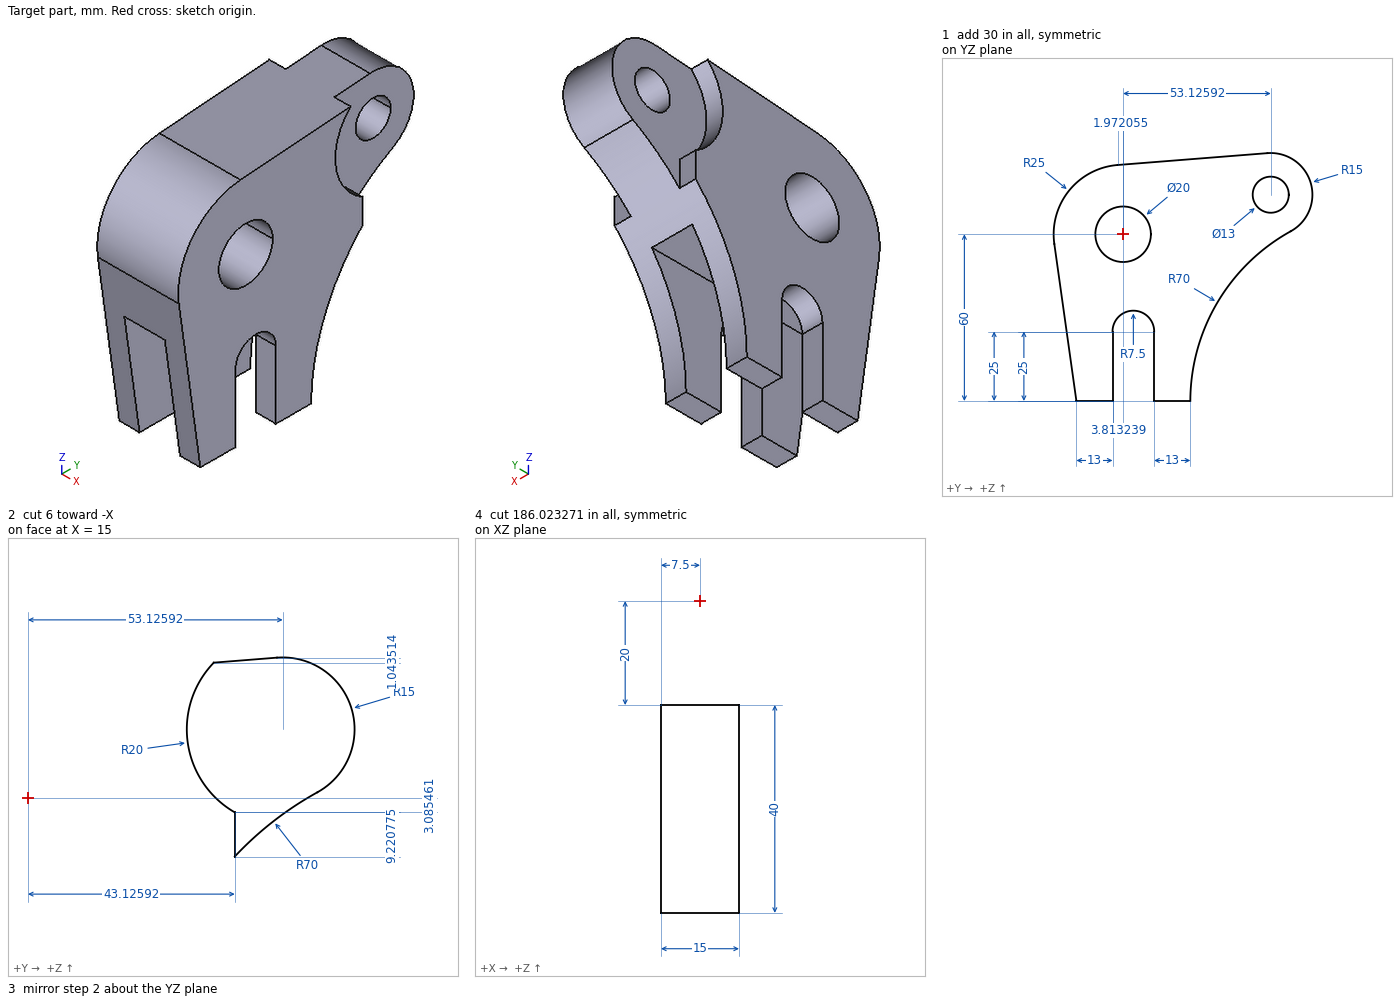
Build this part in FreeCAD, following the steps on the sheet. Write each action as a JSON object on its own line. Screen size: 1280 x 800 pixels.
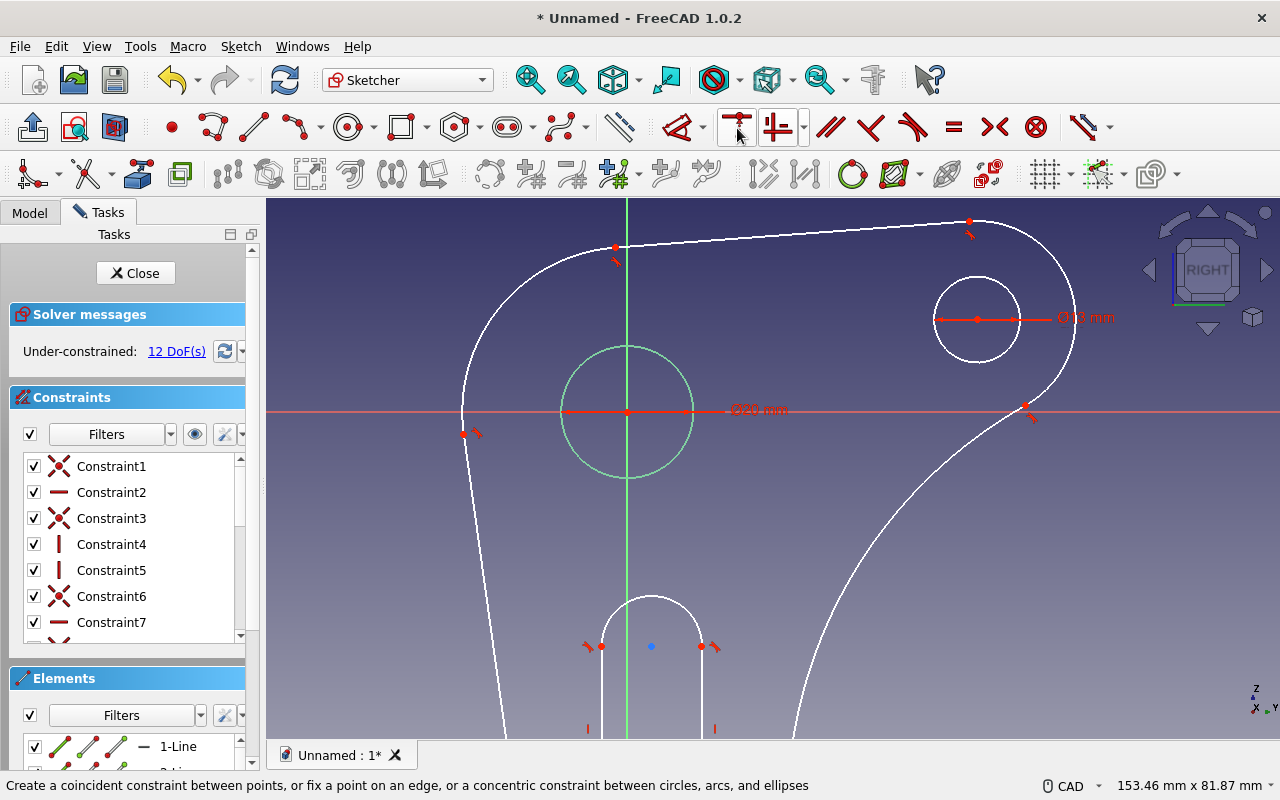
{"action": "left_click", "coordinate": [539, 273]}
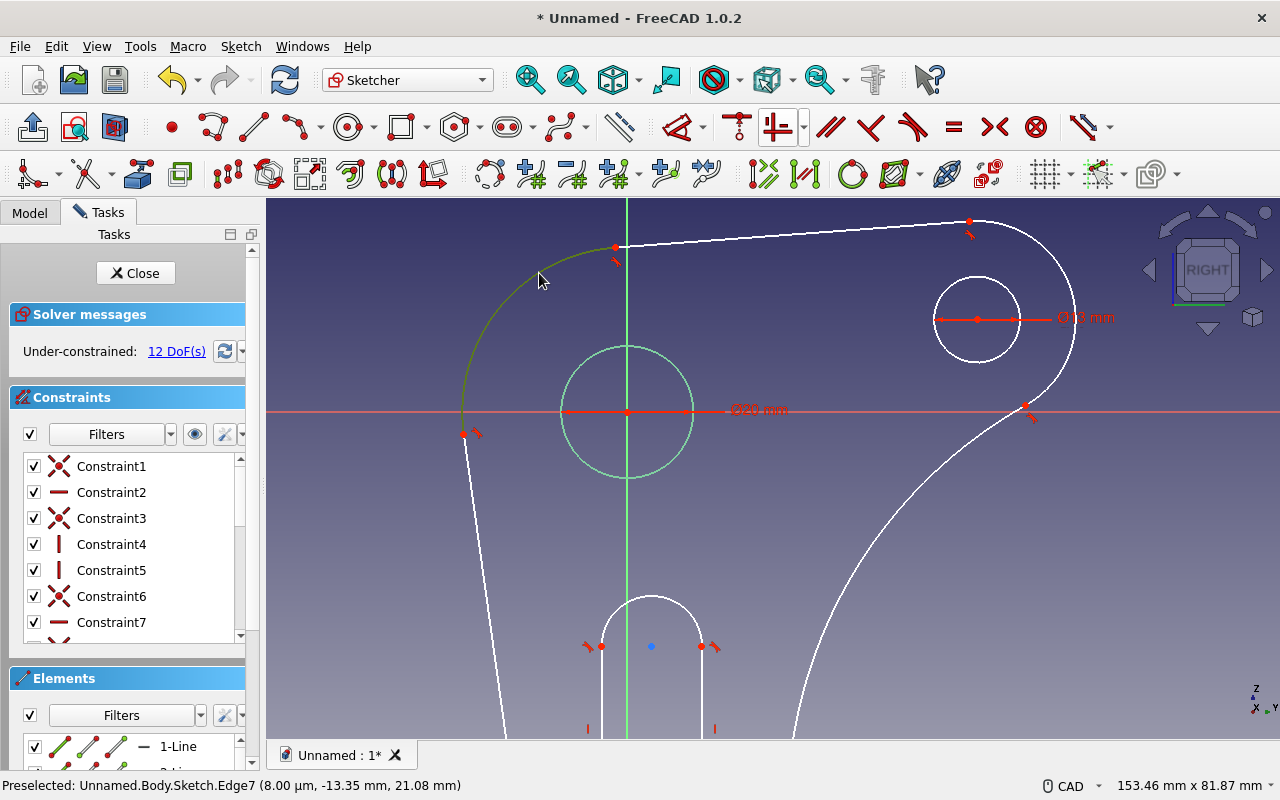
{"action": "left_click", "coordinate": [702, 128]}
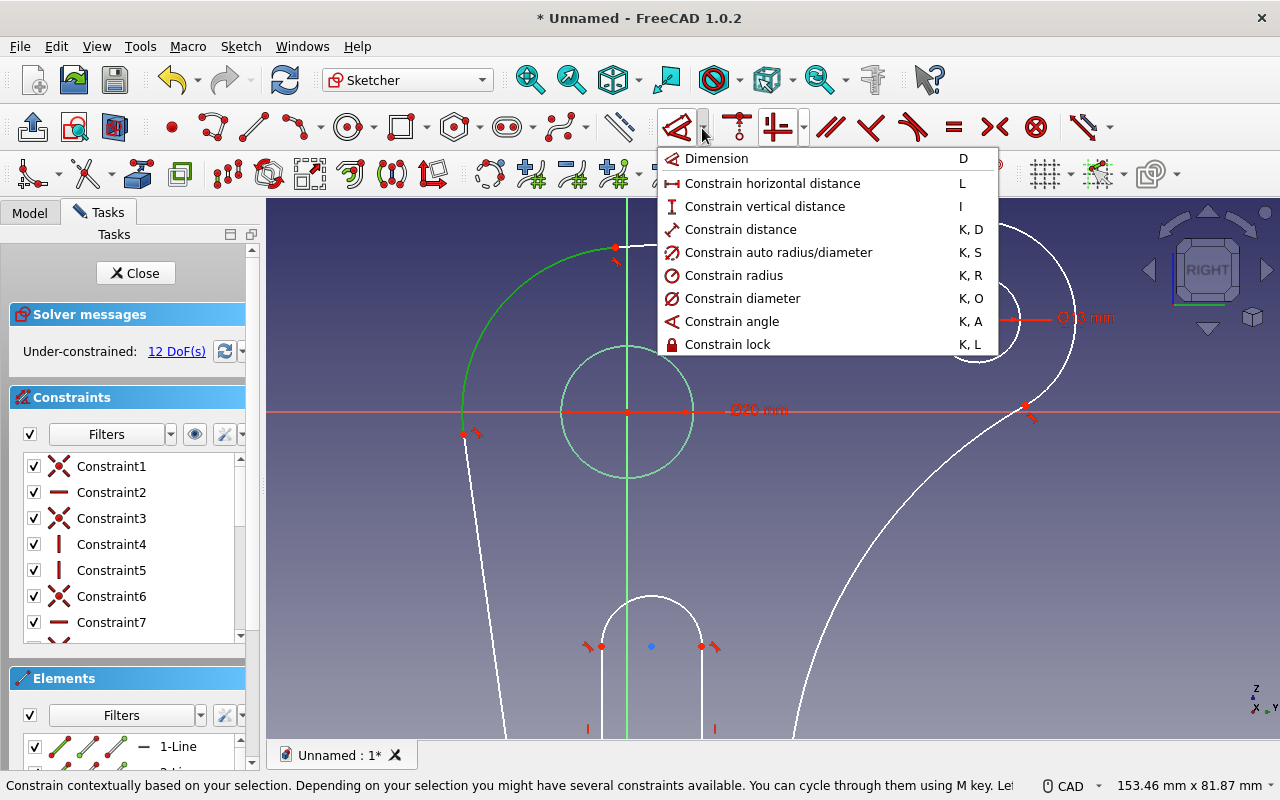
{"action": "left_click", "coordinate": [828, 276]}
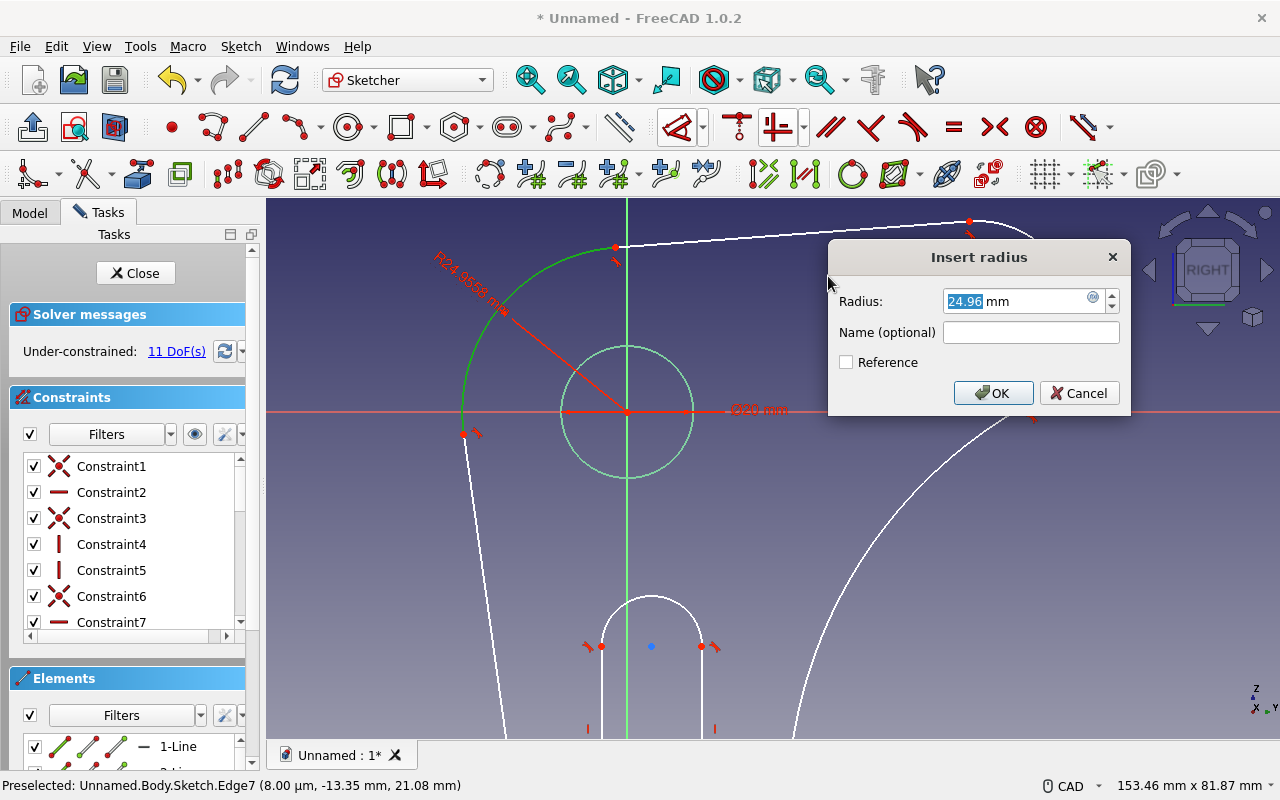
{"action": "type", "text": "25"}
{"action": "key", "text": "Return"}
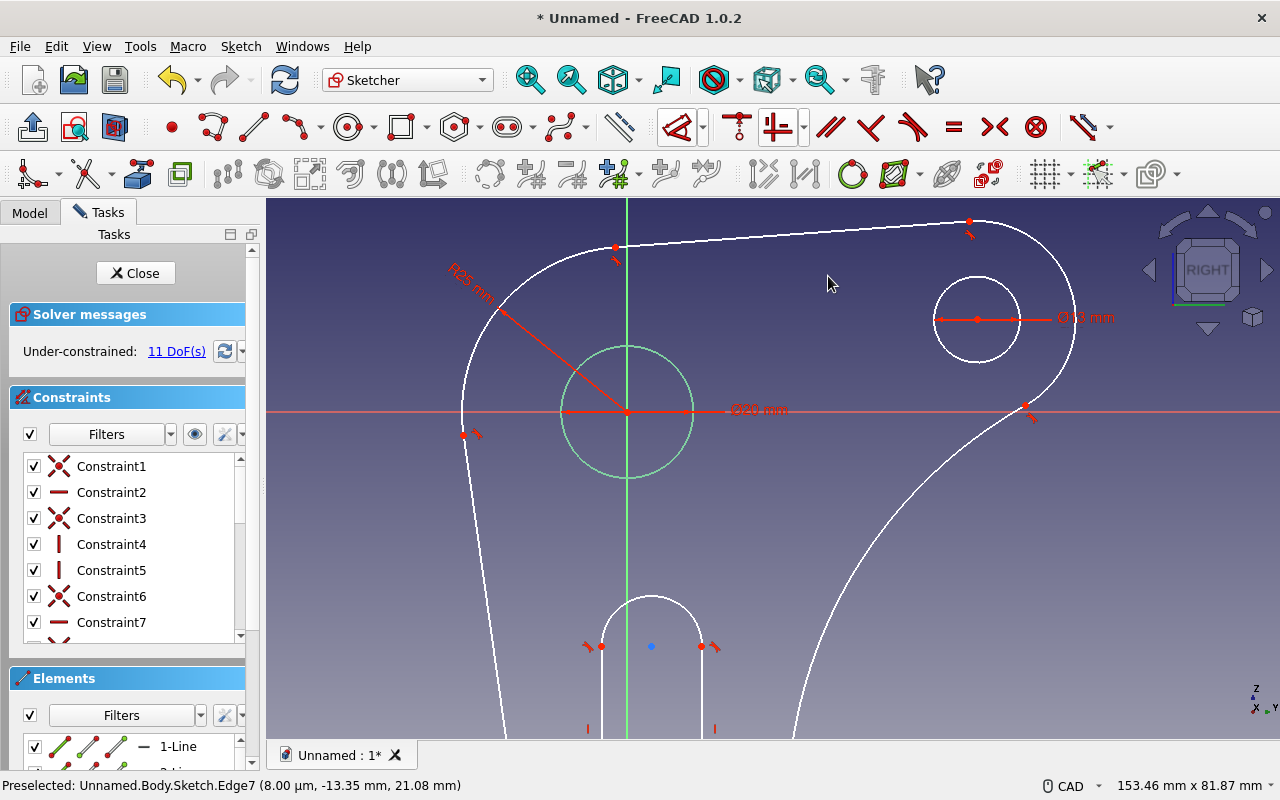
{"action": "left_click", "coordinate": [681, 606]}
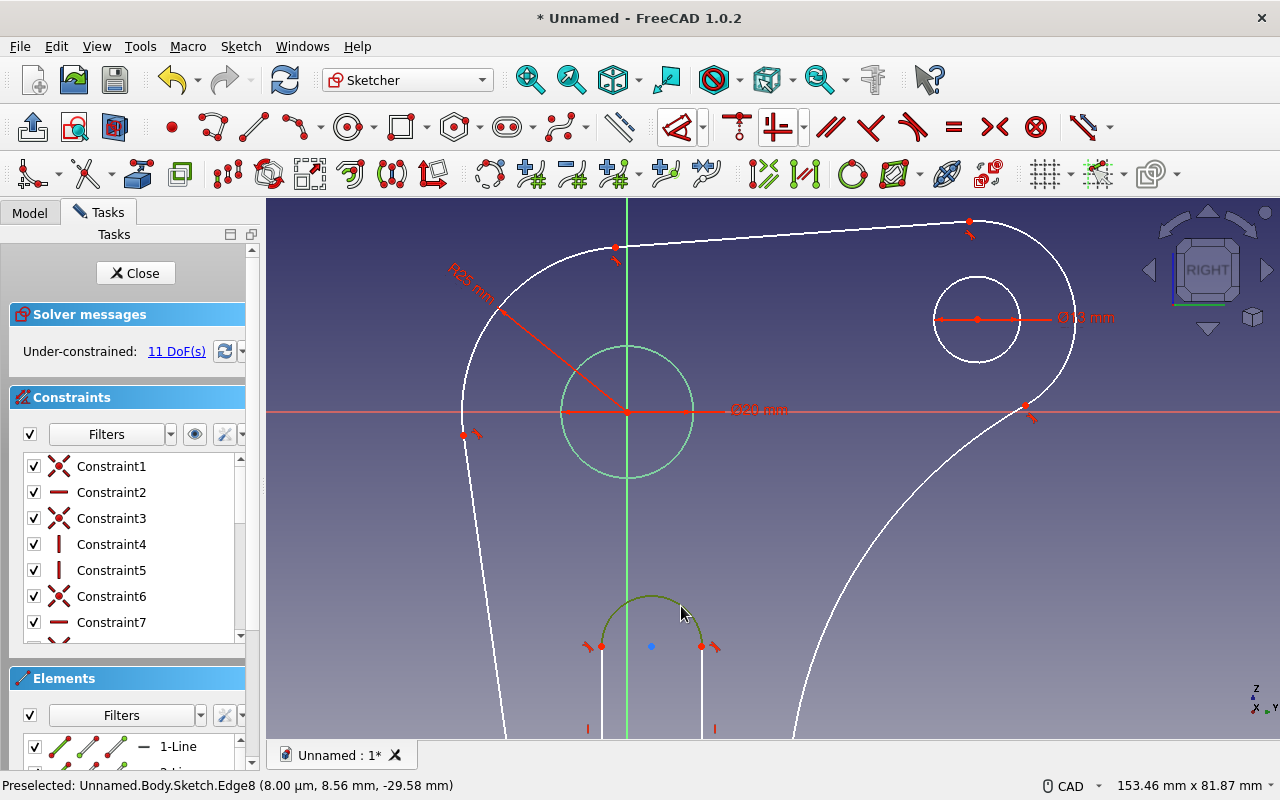
{"action": "key", "text": "k r"}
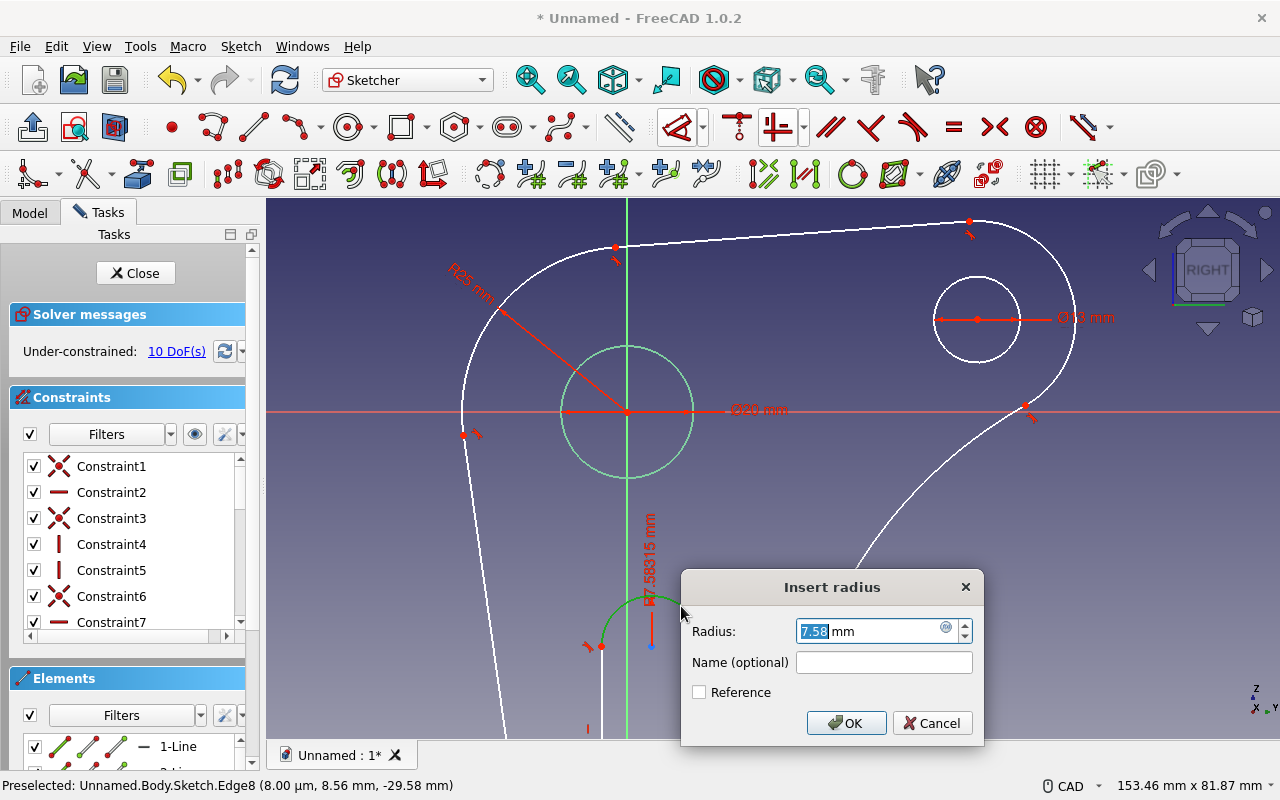
{"action": "type", "text": "7.5"}
{"action": "key", "text": "Return"}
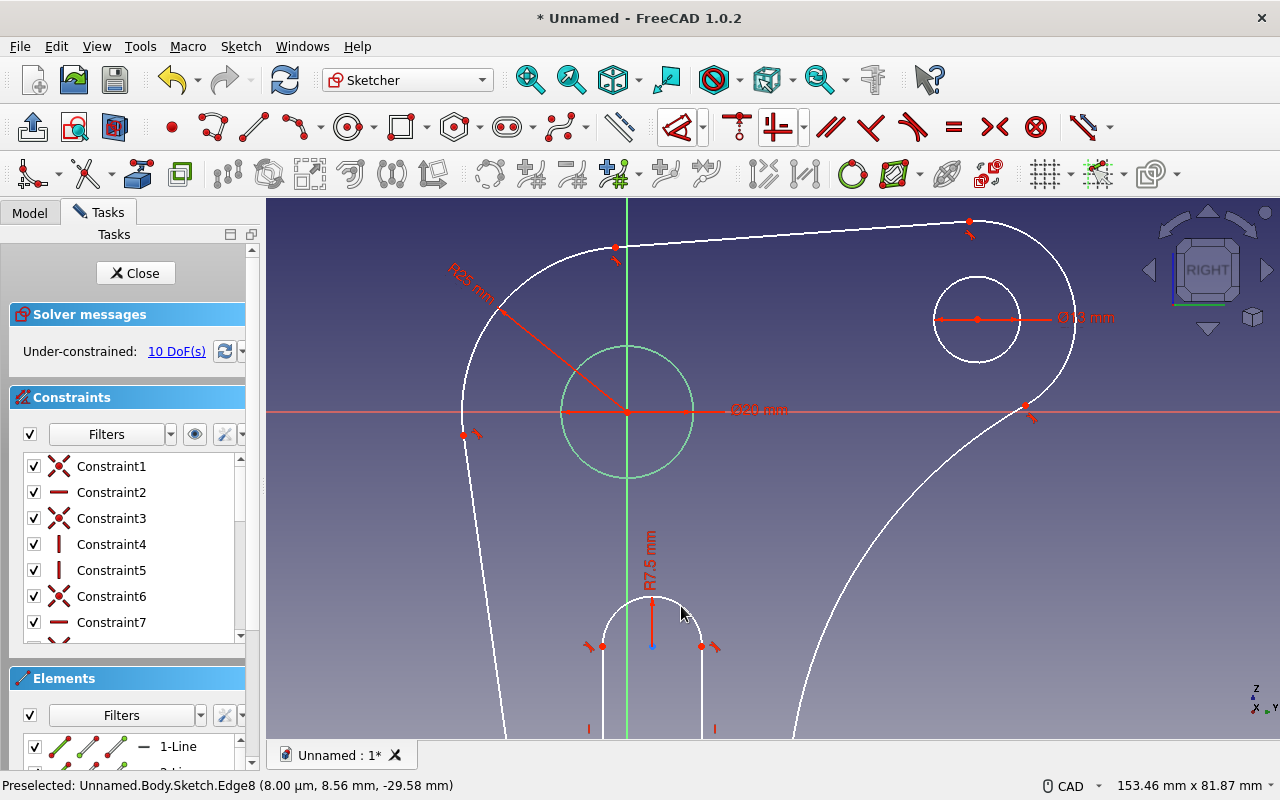
{"action": "left_click", "coordinate": [910, 497]}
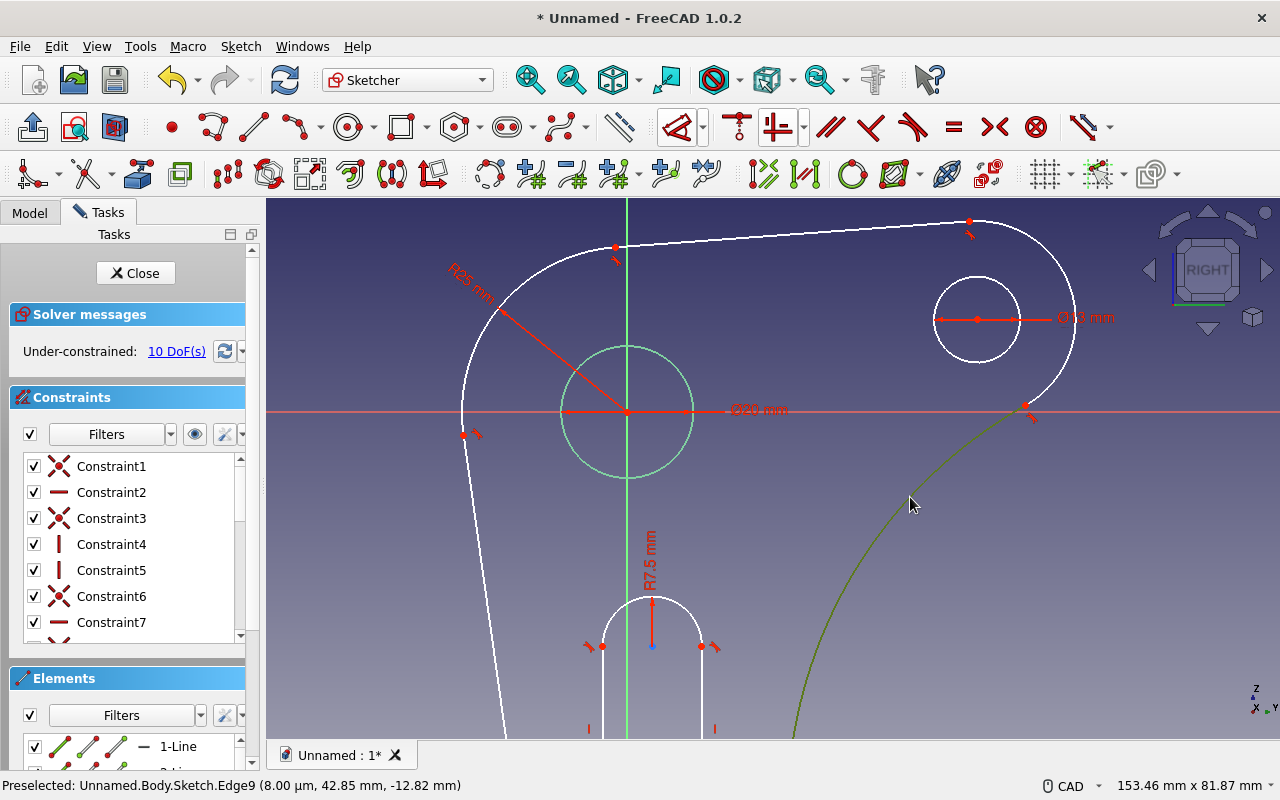
{"action": "key", "text": "k r"}